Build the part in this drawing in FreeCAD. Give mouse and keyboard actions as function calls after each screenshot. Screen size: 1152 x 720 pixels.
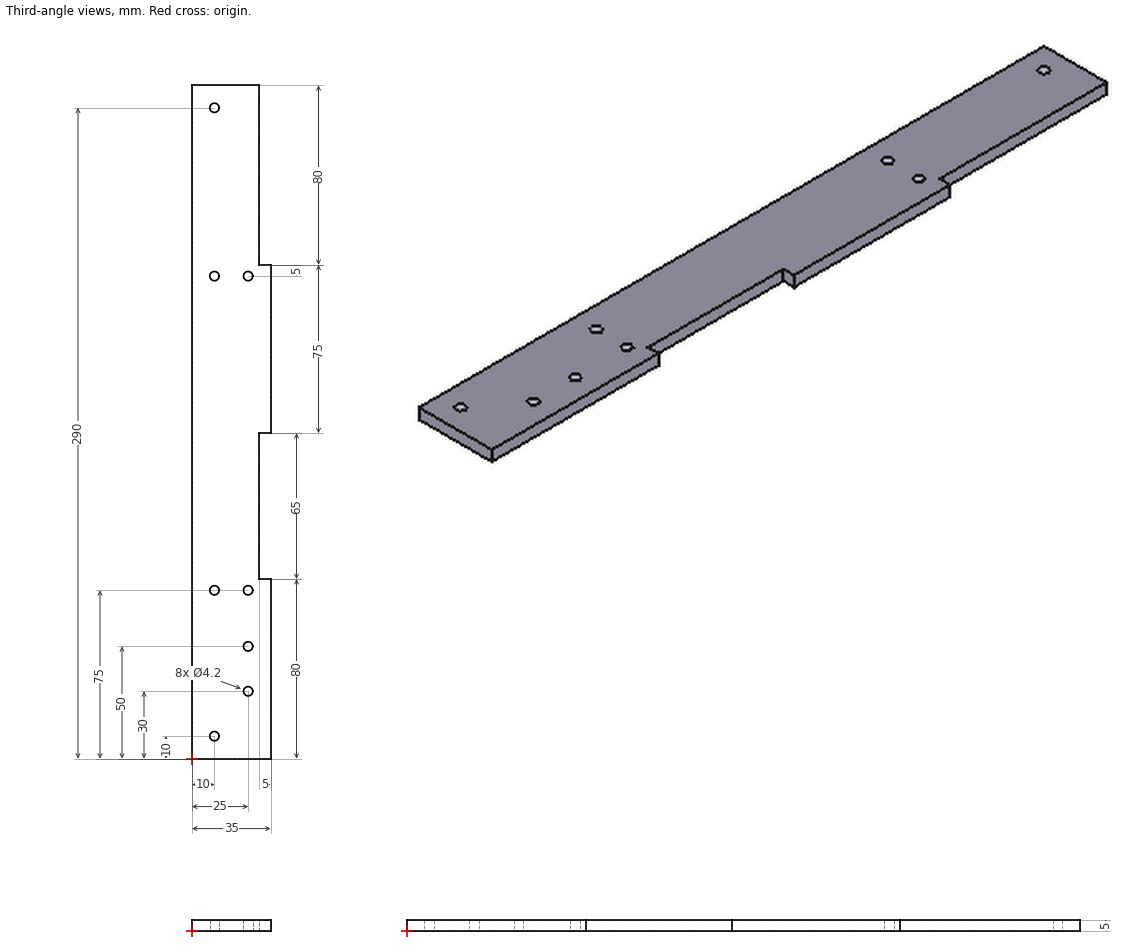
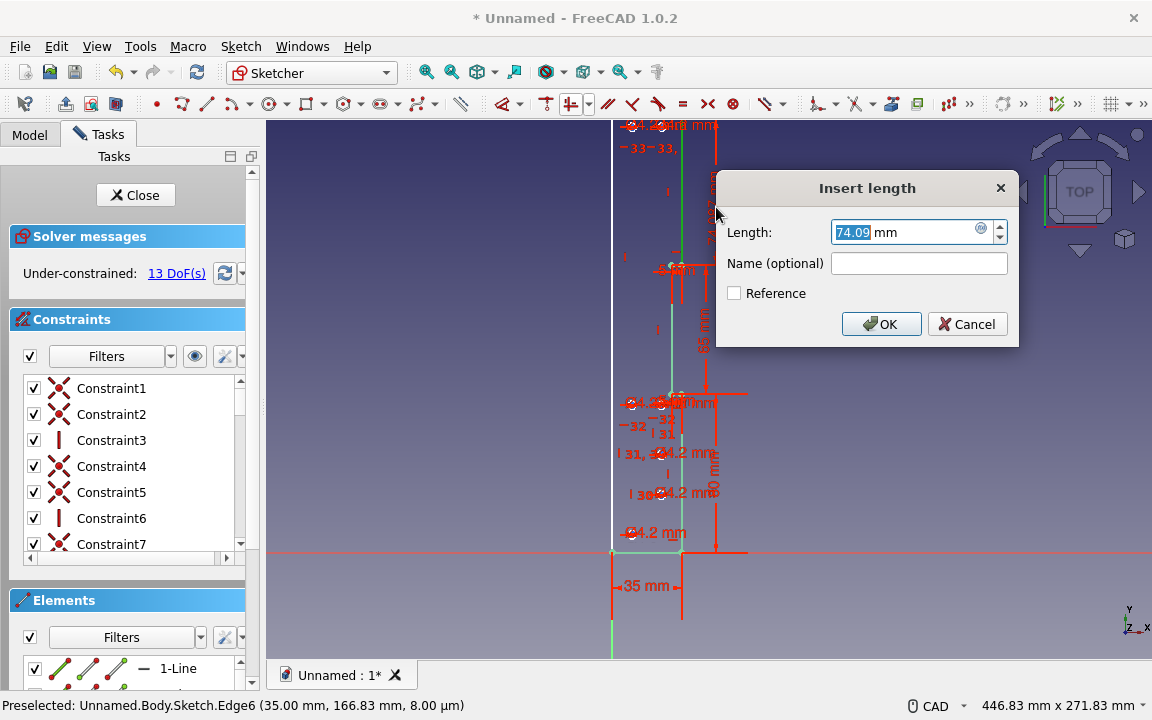
text(75)
key(Return)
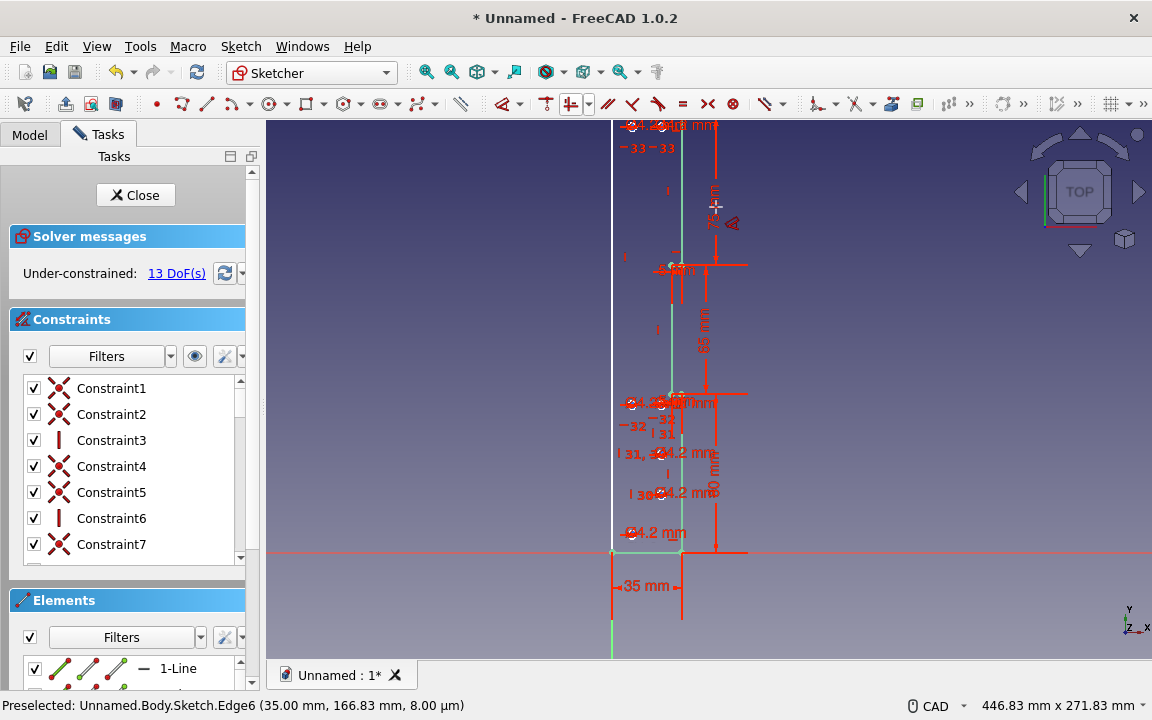
scroll(633, 553, down, 3)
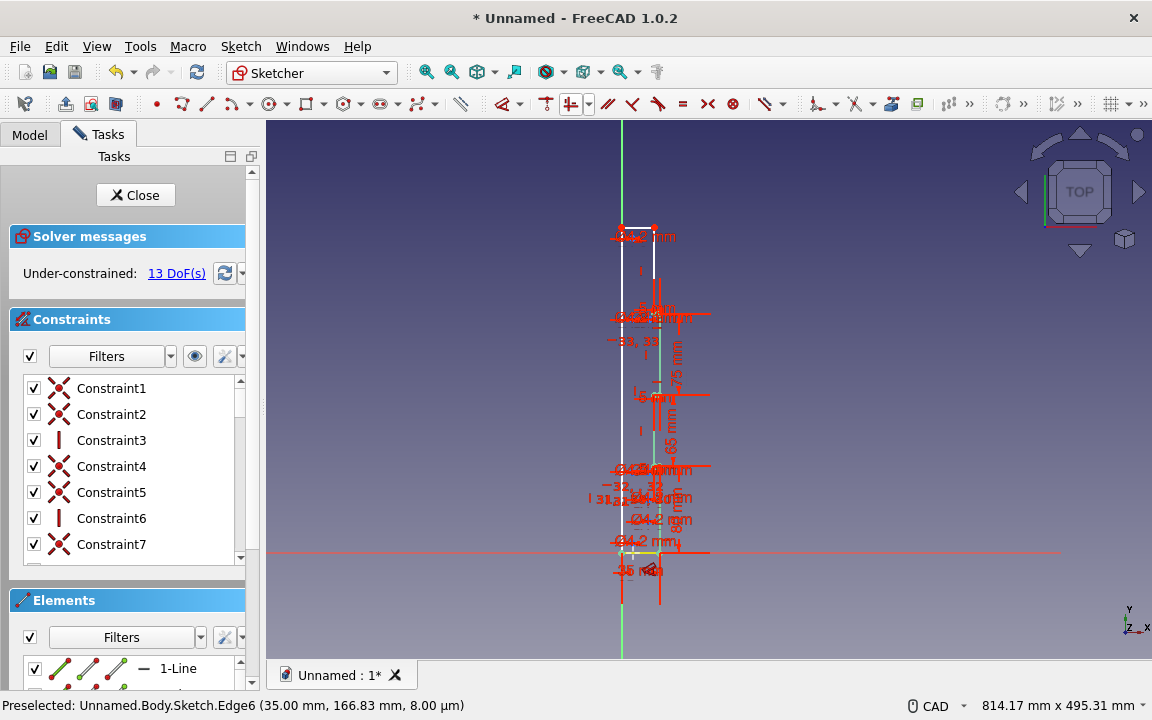
click(654, 288)
click(688, 271)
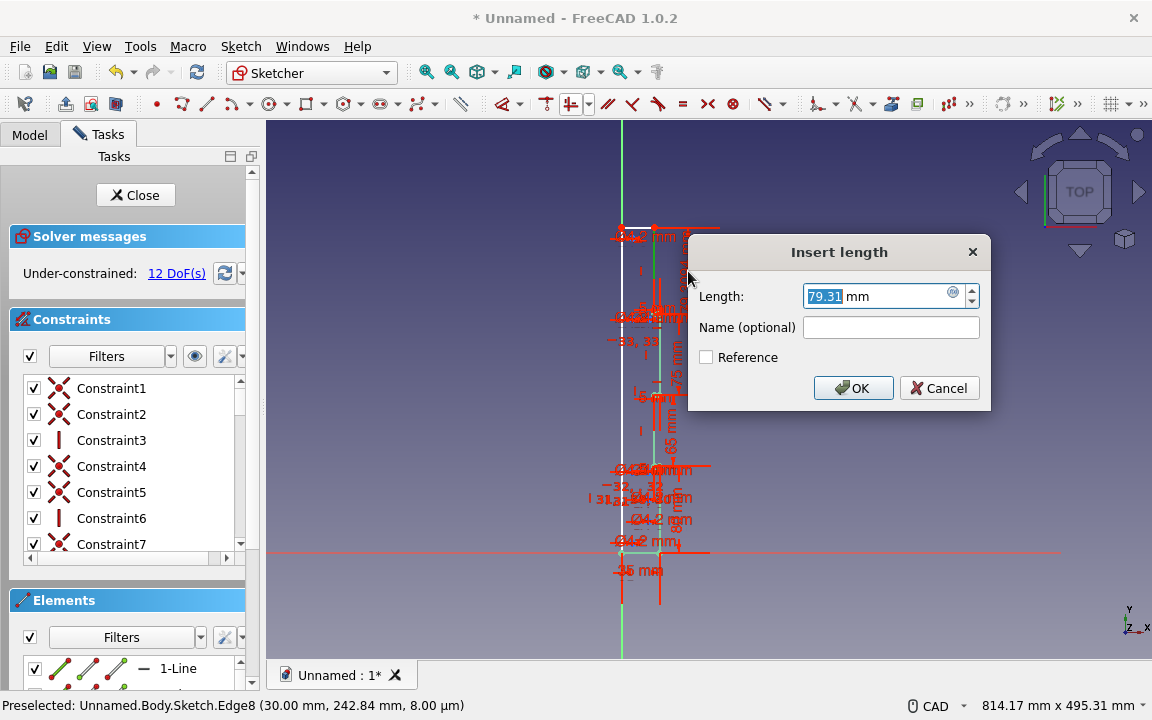
text(80)
key(Return)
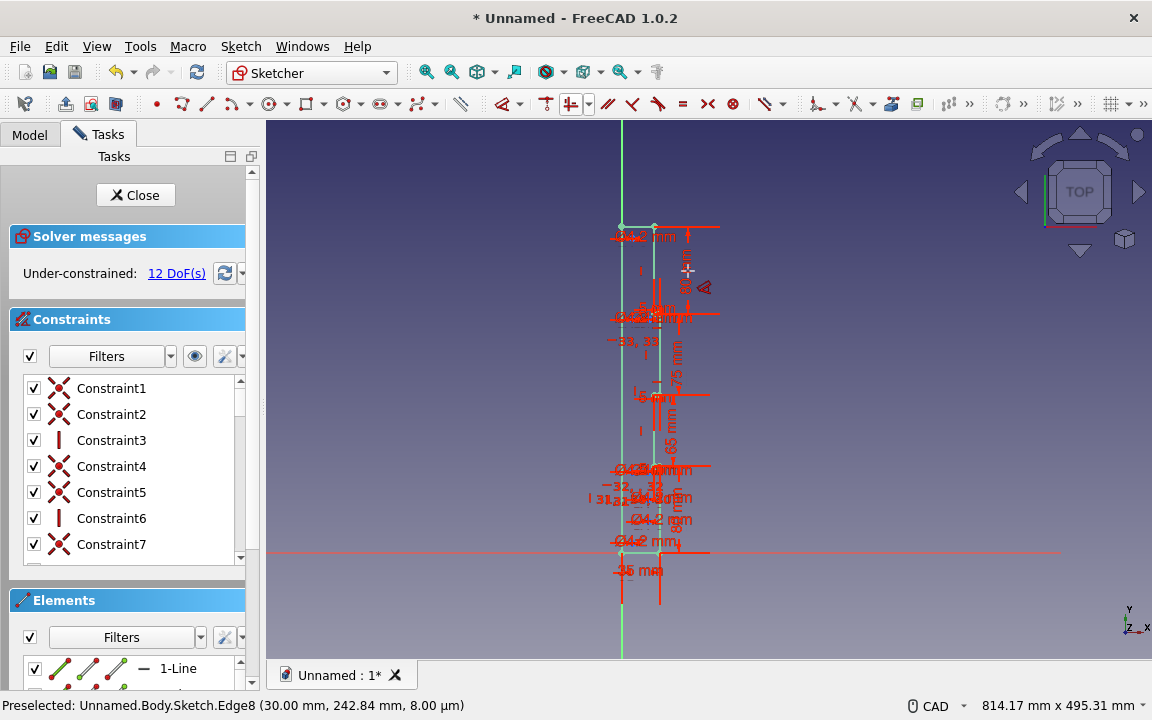
scroll(649, 522, up, 2)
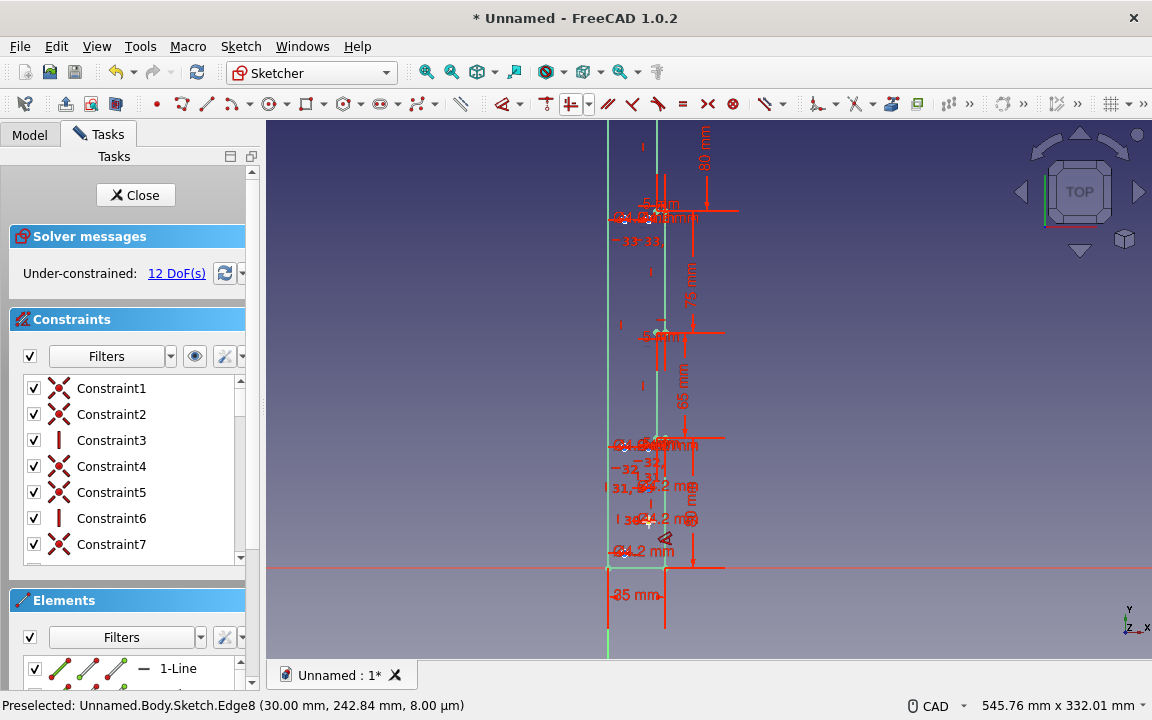
click(649, 521)
click(628, 626)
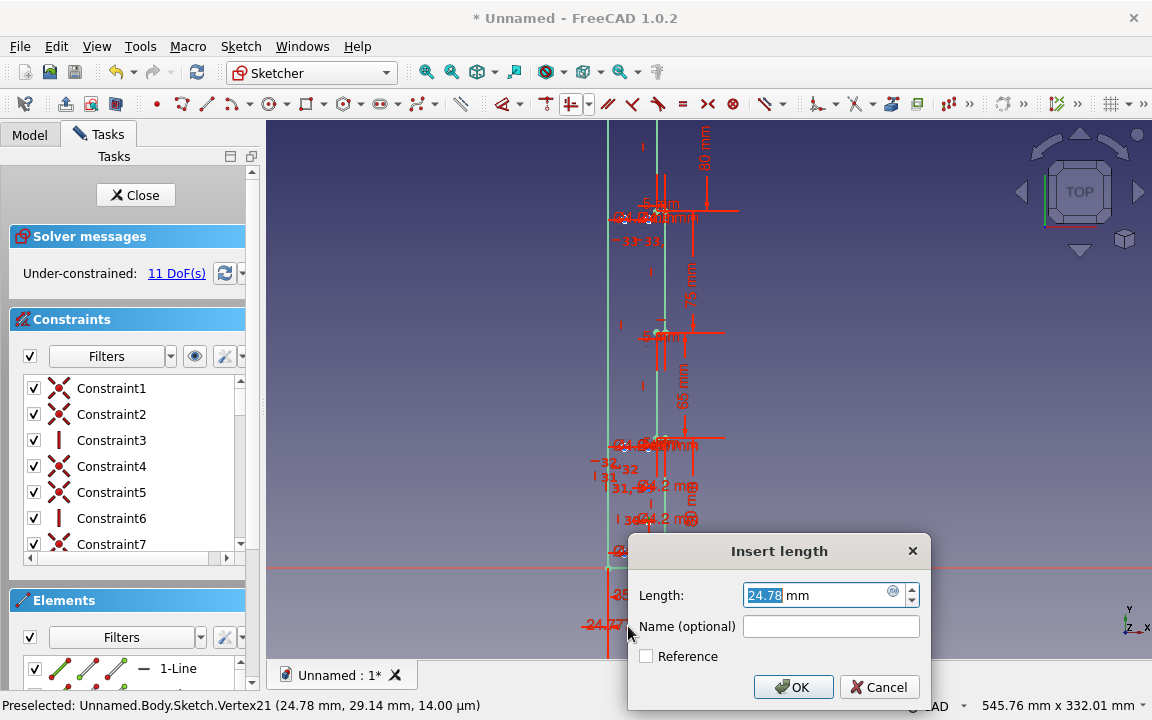
text(25)
key(Return)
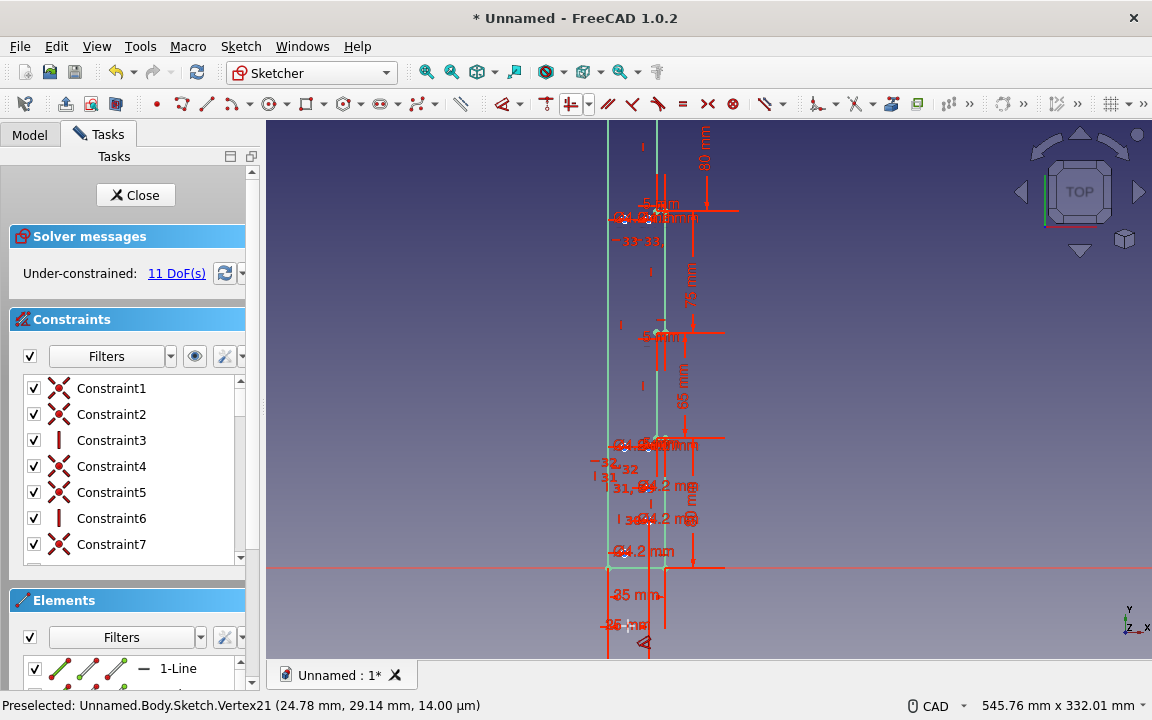
click(649, 521)
click(574, 545)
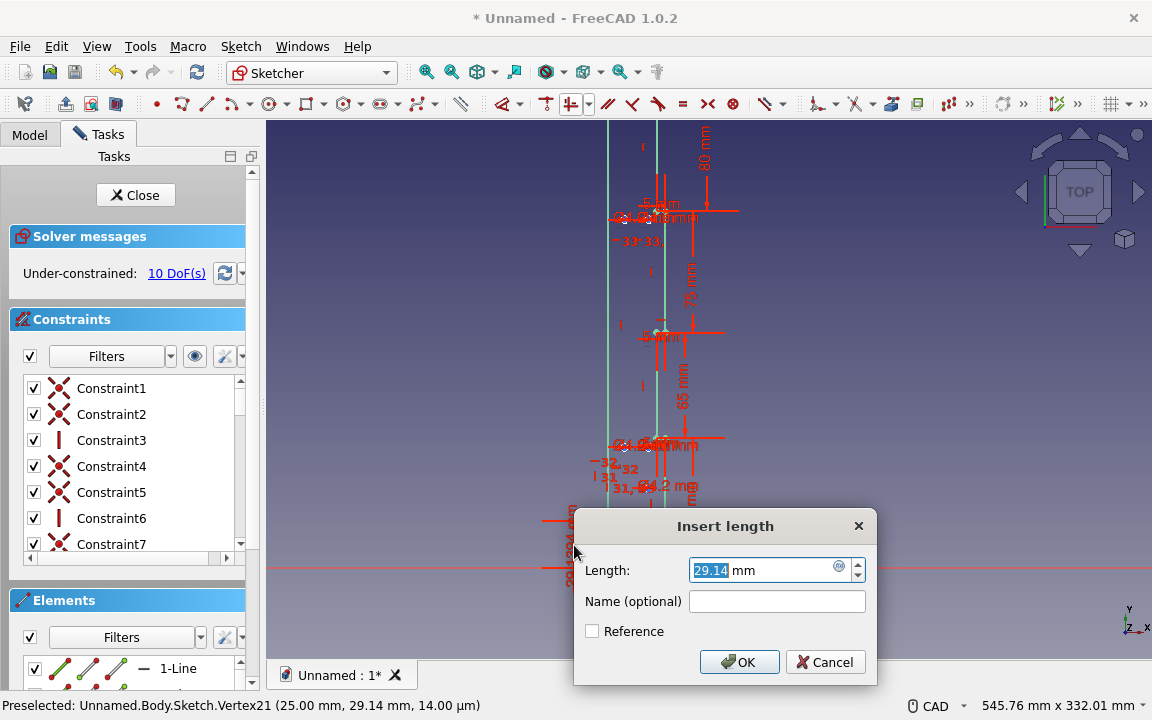
text(30)
key(Return)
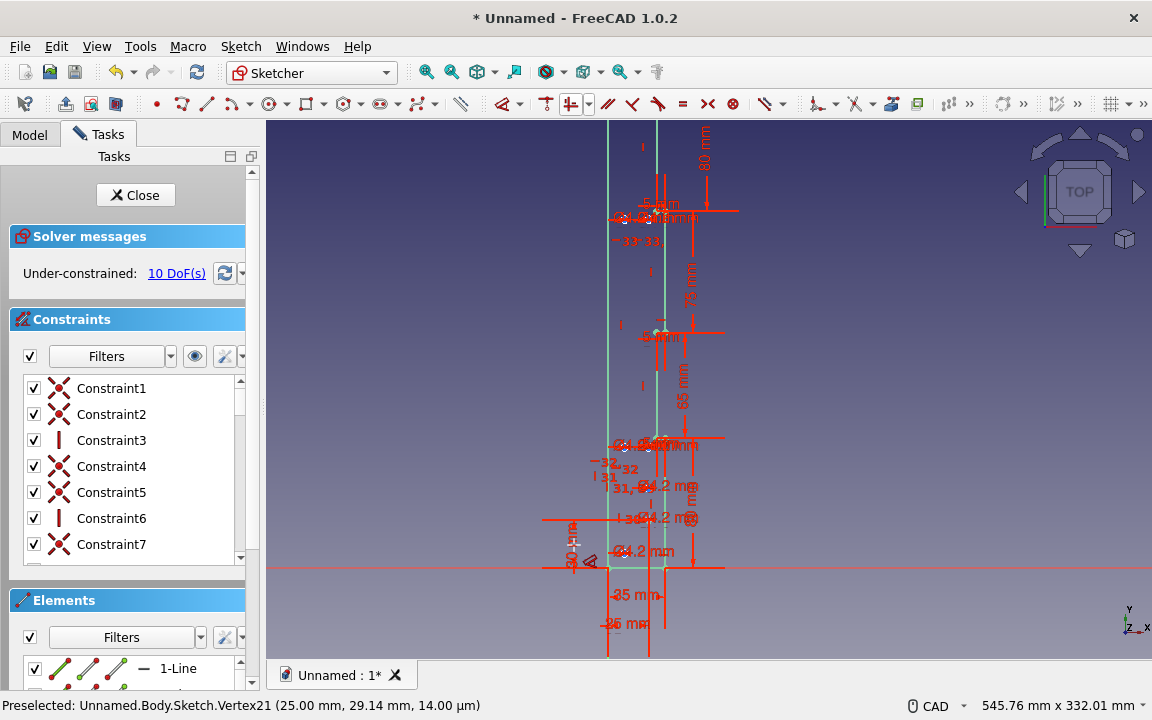
click(649, 488)
click(574, 510)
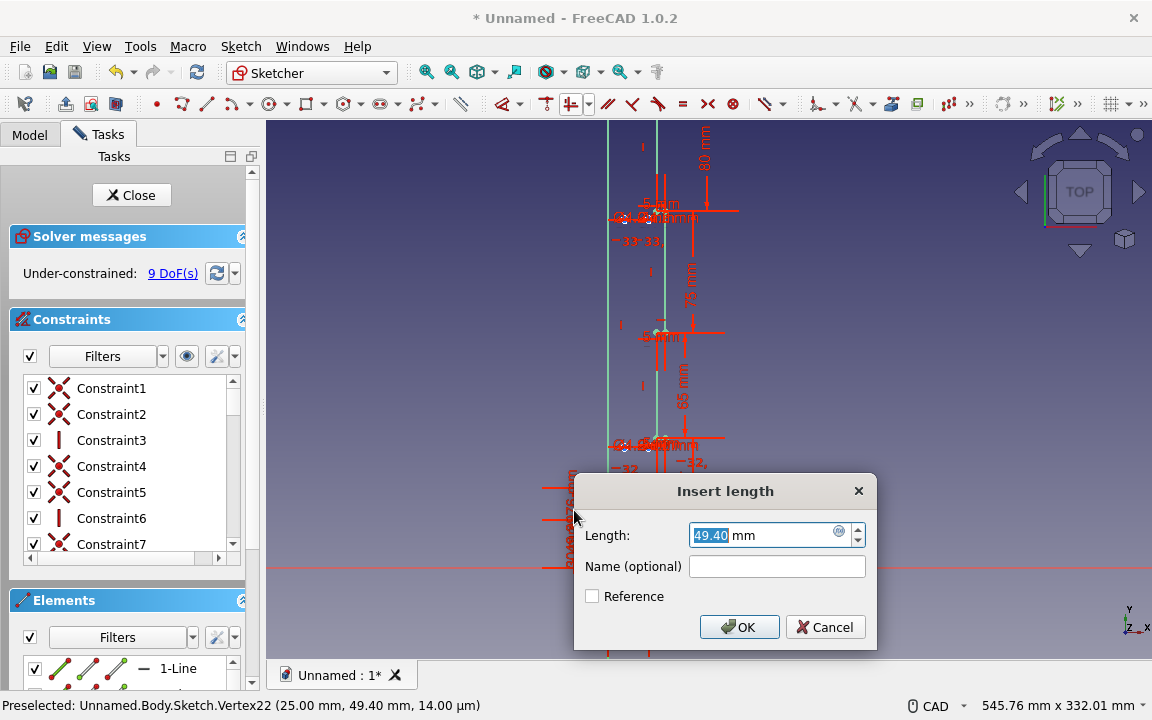
text(50)
key(Return)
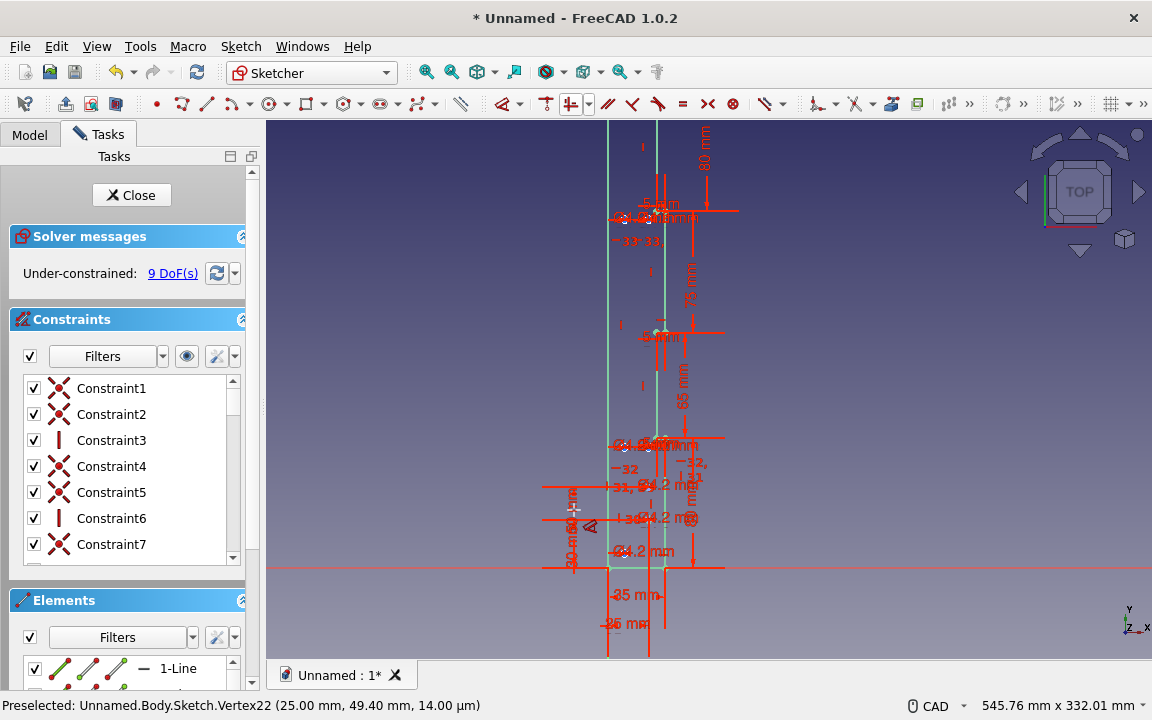
click(649, 447)
click(574, 480)